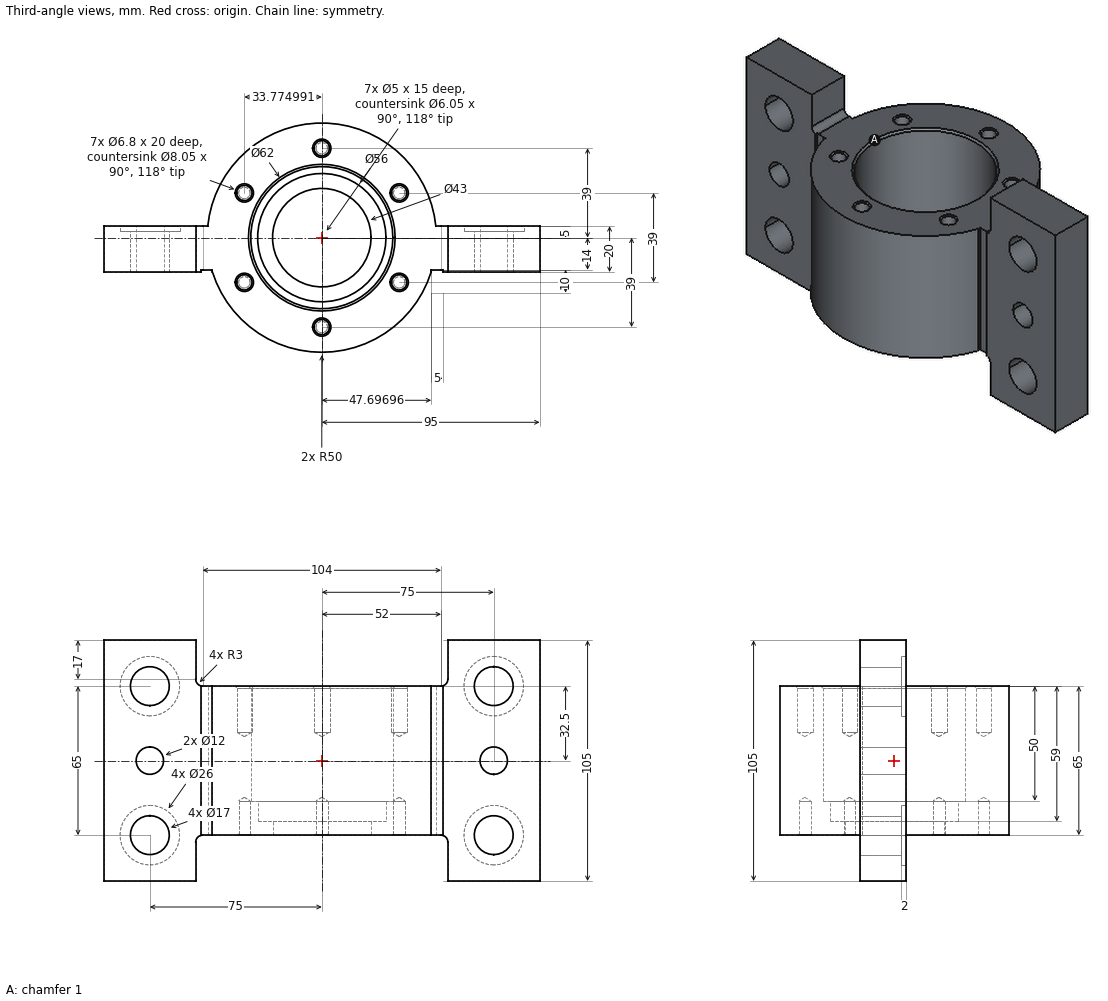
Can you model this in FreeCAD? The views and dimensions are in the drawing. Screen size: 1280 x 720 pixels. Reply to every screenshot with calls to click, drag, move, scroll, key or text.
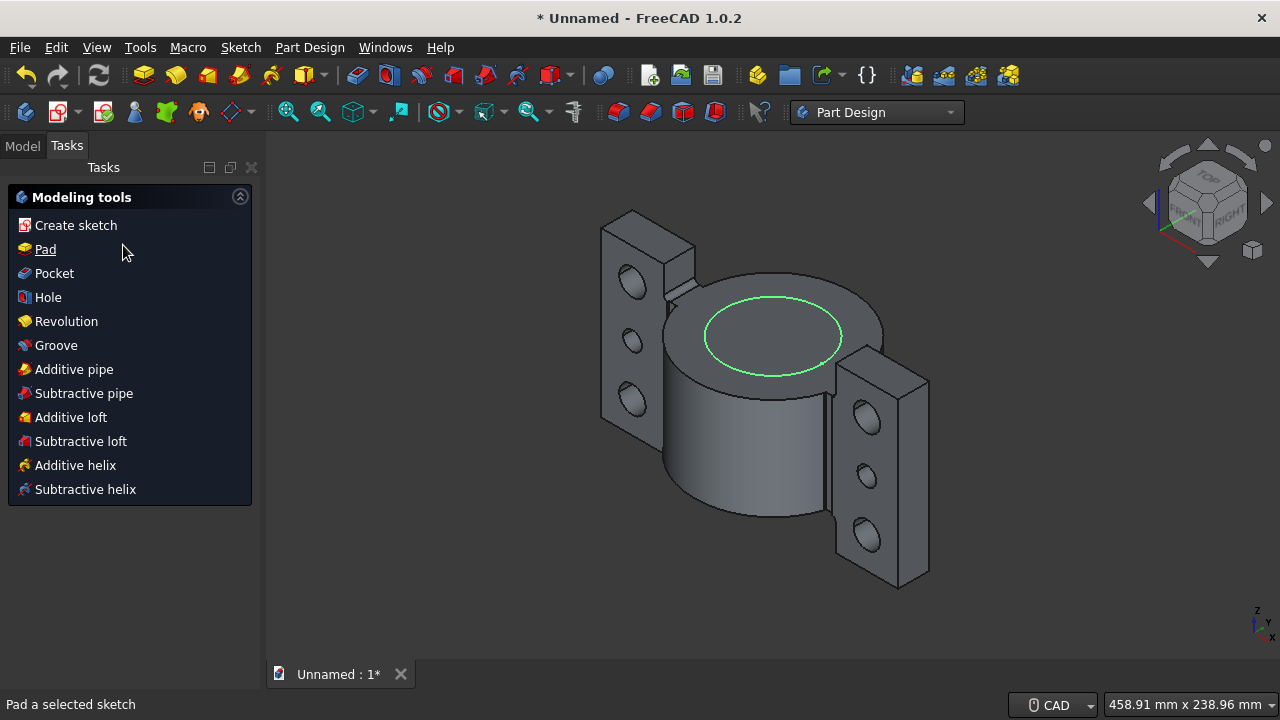
click(358, 76)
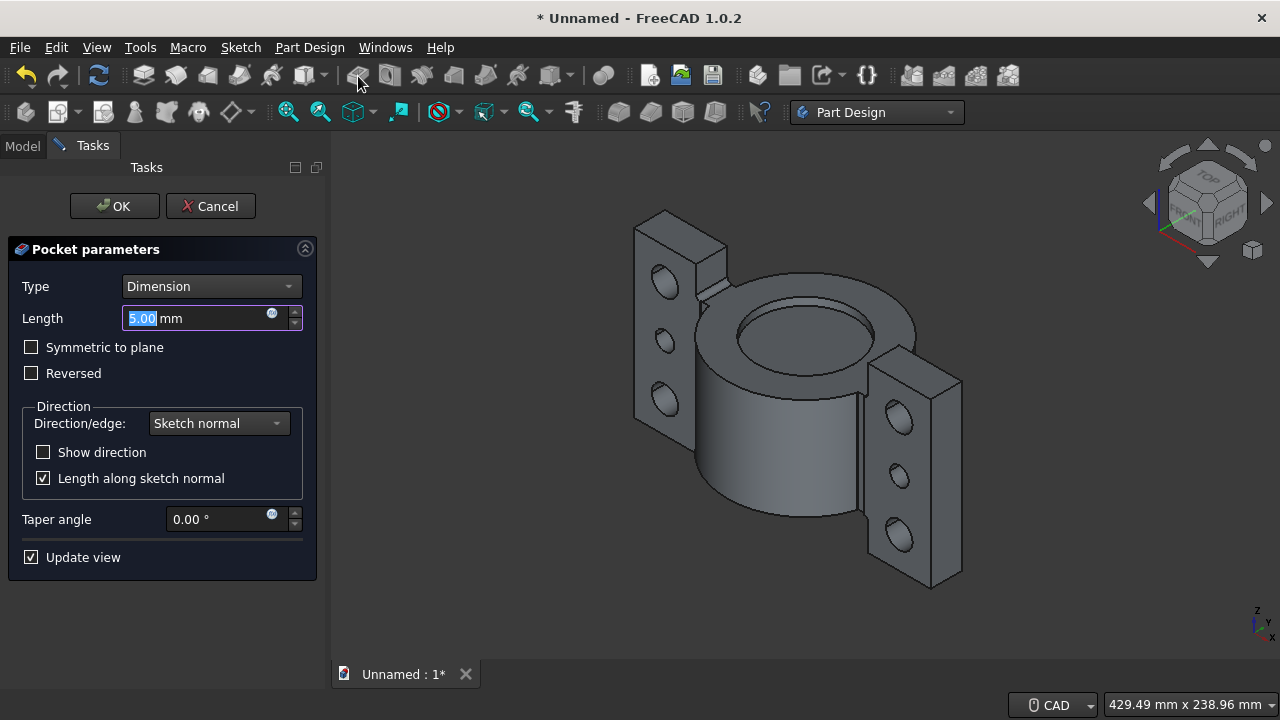
text(50)
key(Tab)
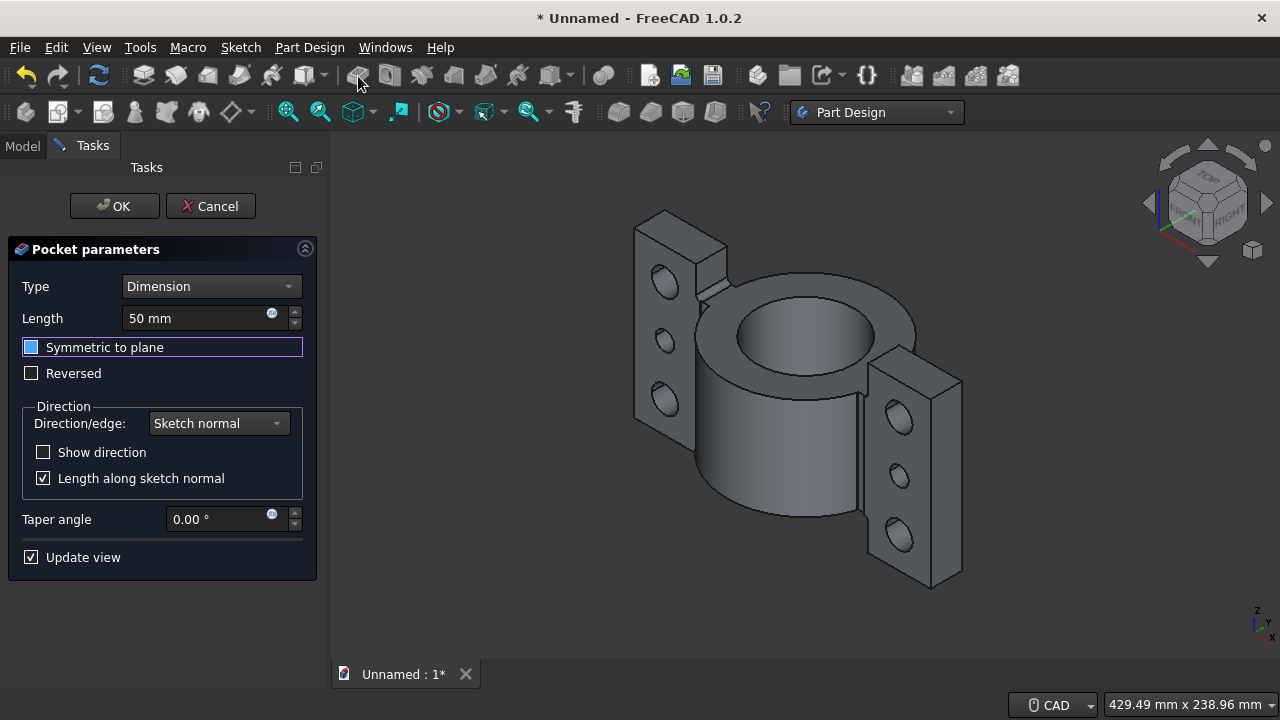
click(115, 206)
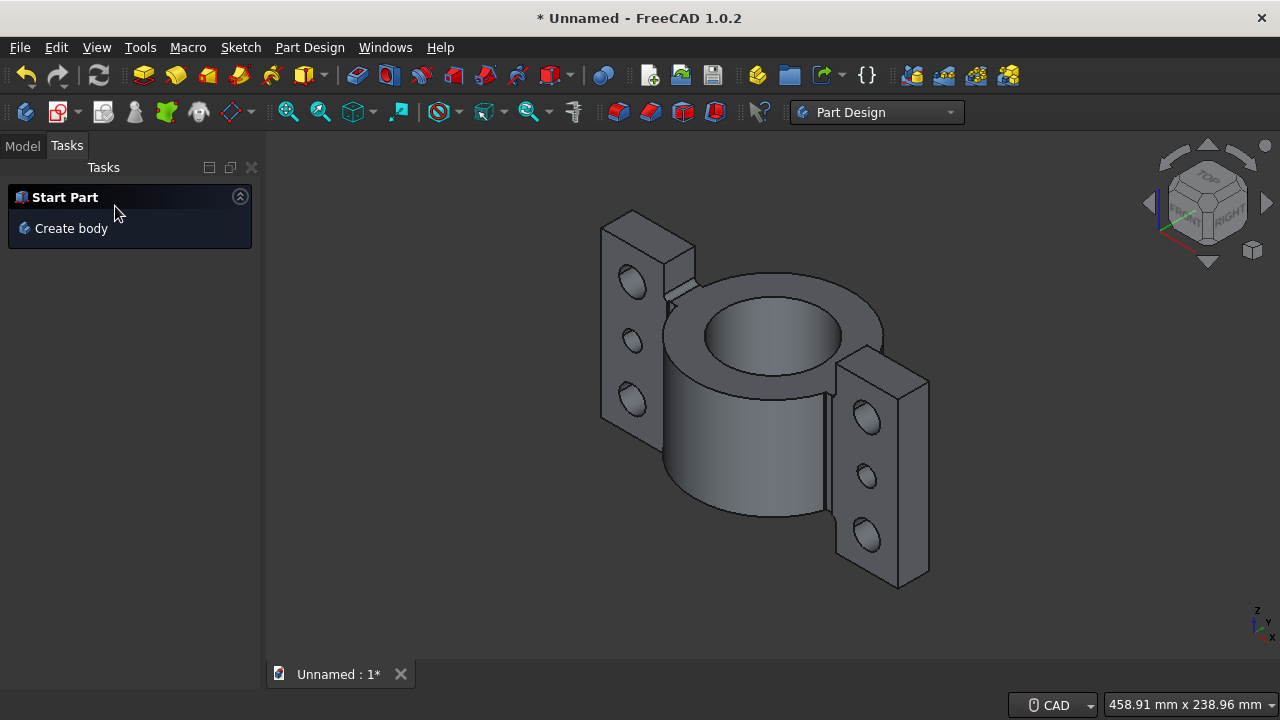
click(771, 283)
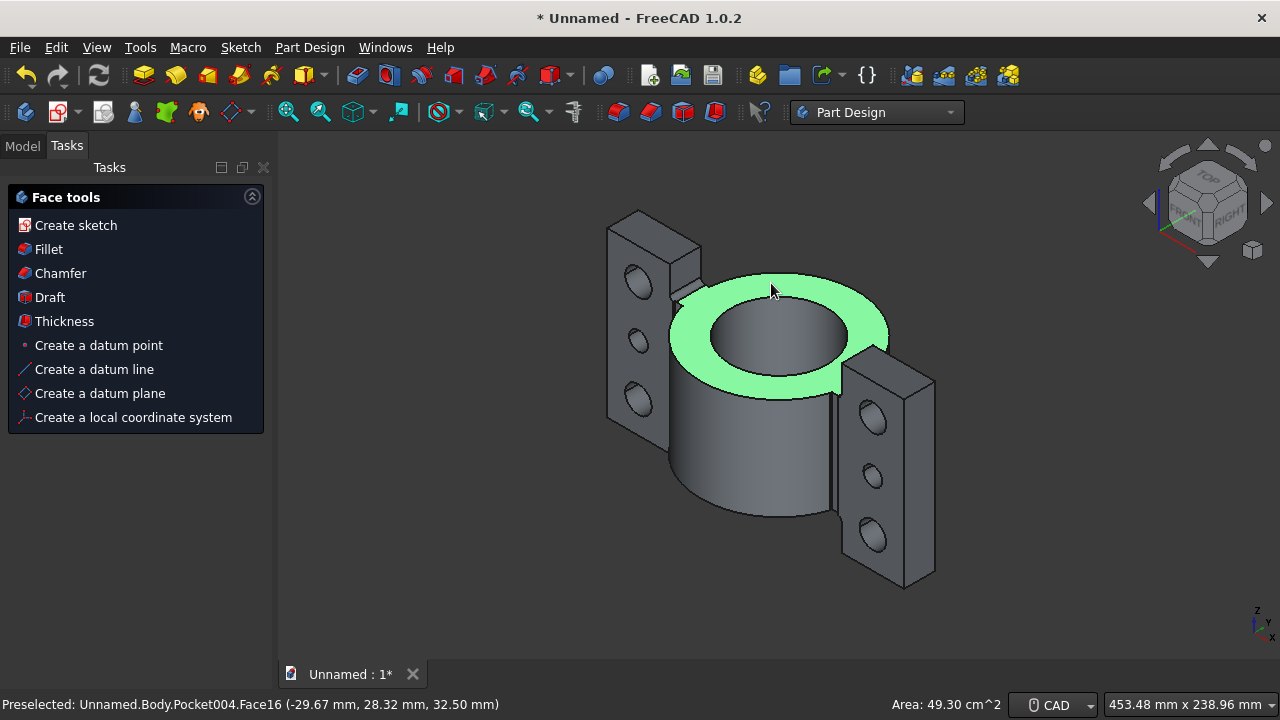
click(58, 112)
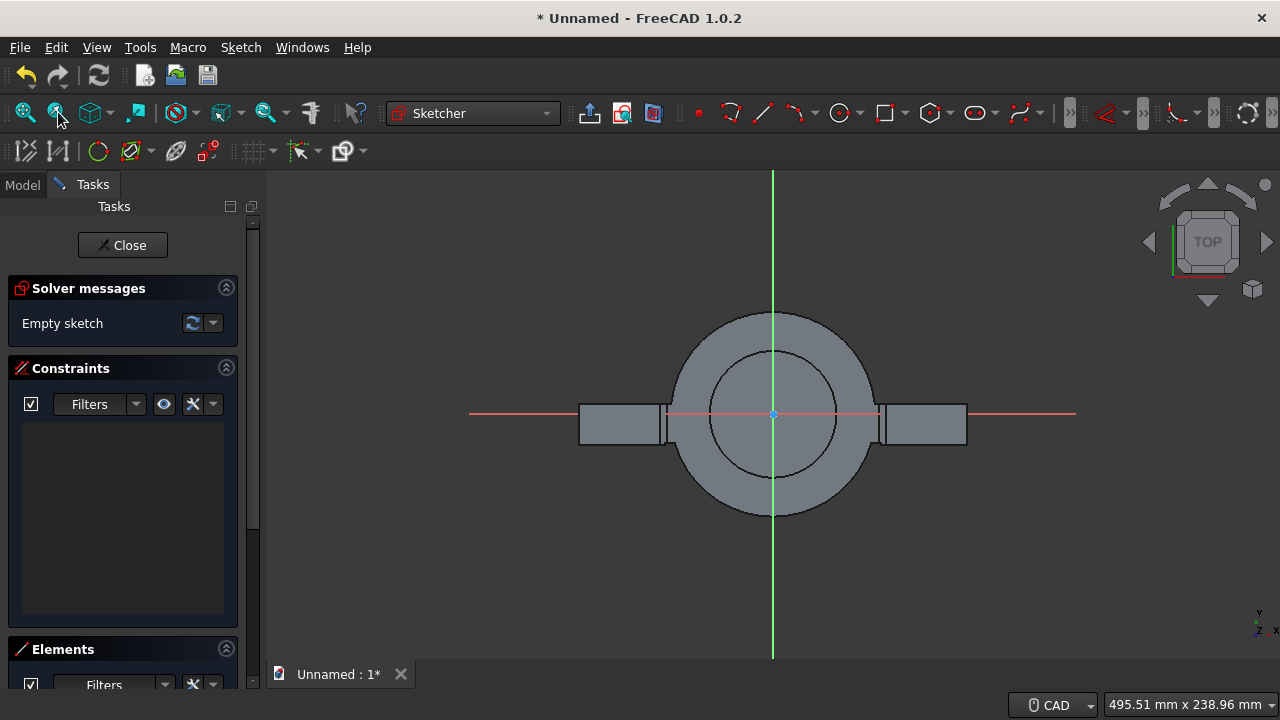
scroll(813, 414, up, 5)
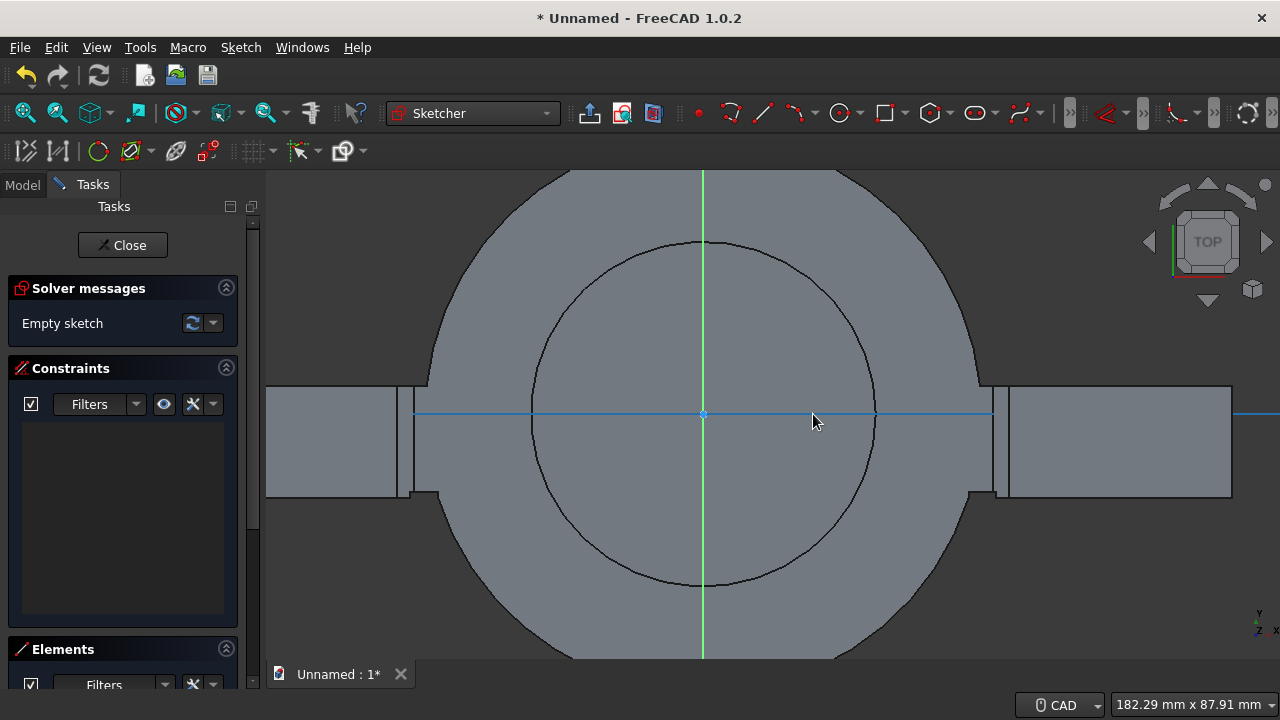
click(840, 114)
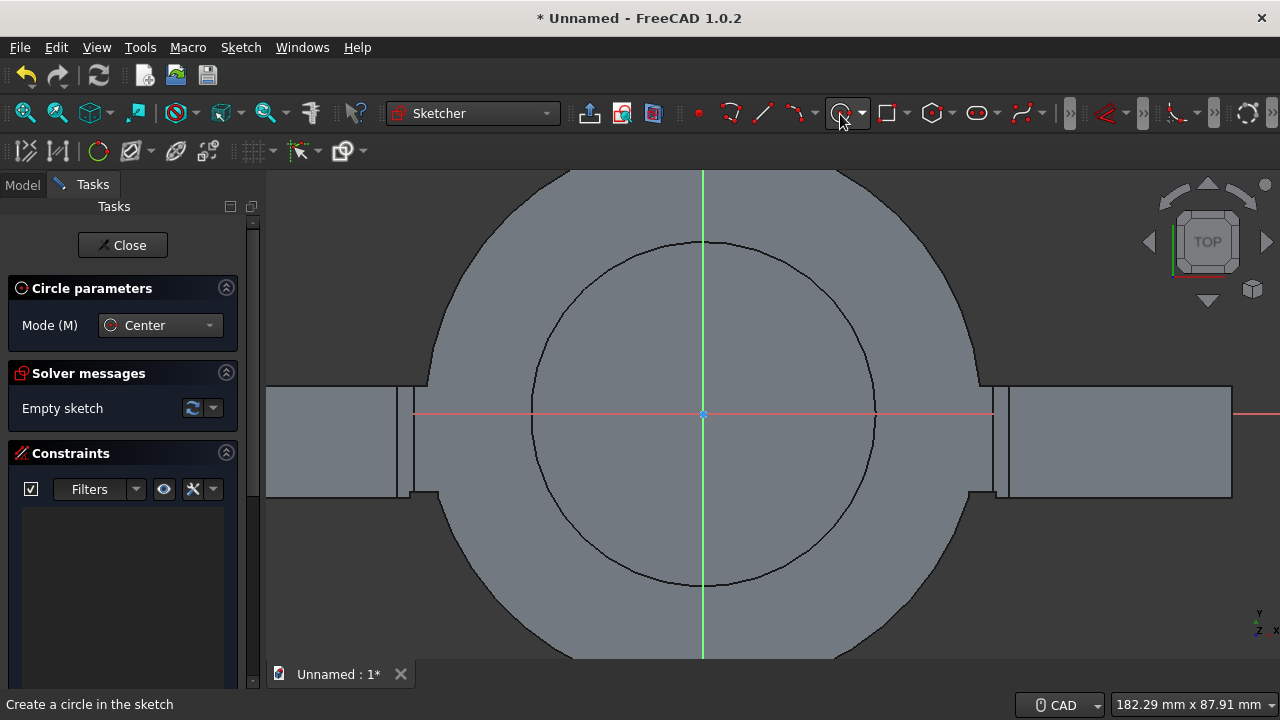
click(703, 414)
click(813, 304)
key(Escape)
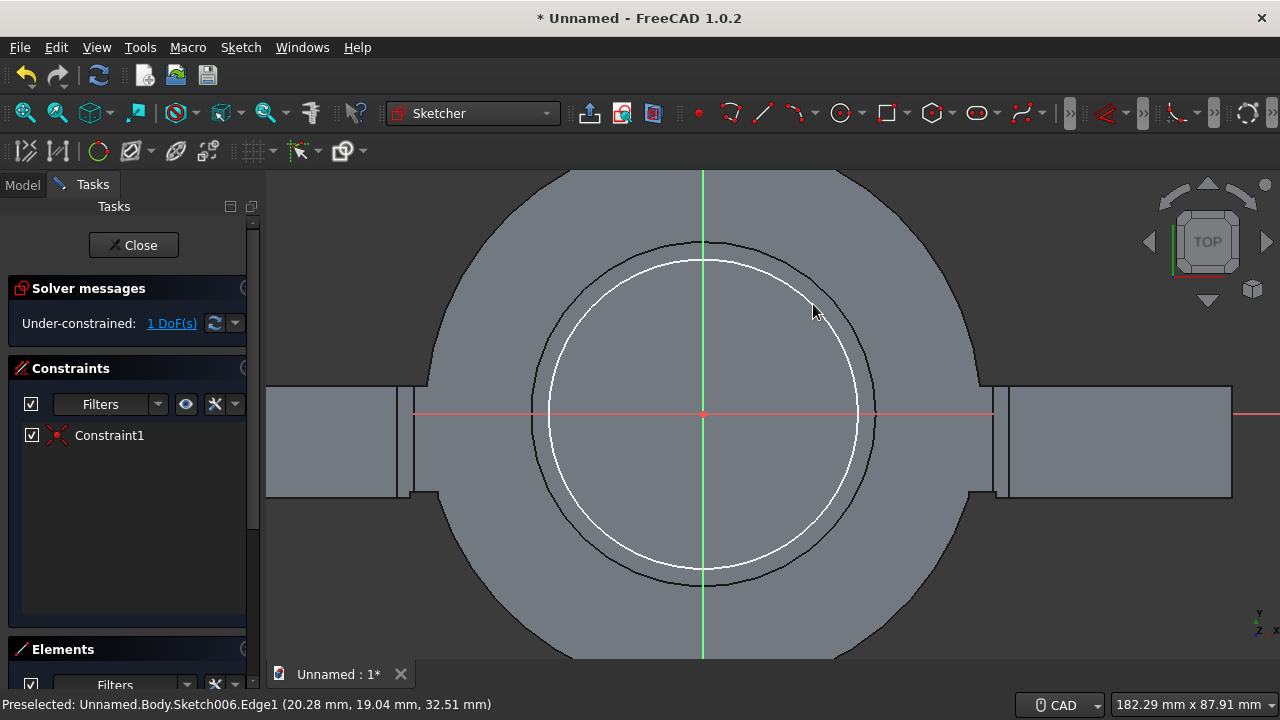
click(1106, 114)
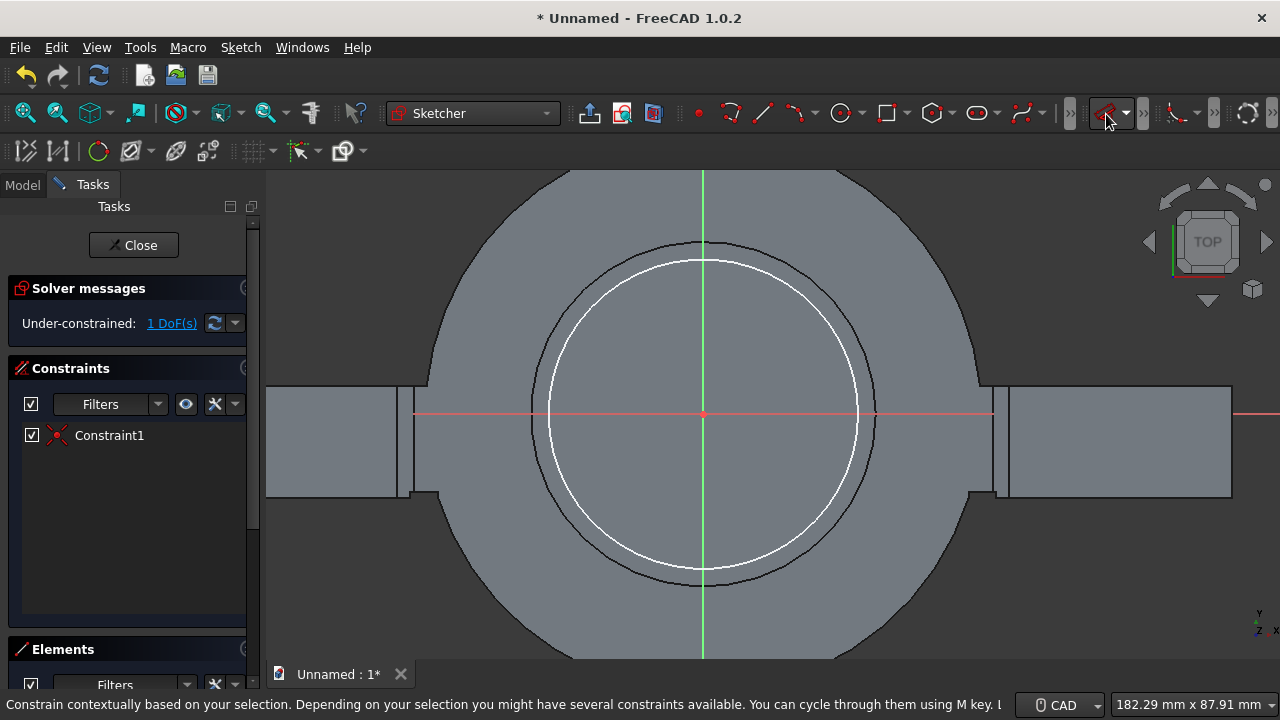
click(812, 304)
click(834, 281)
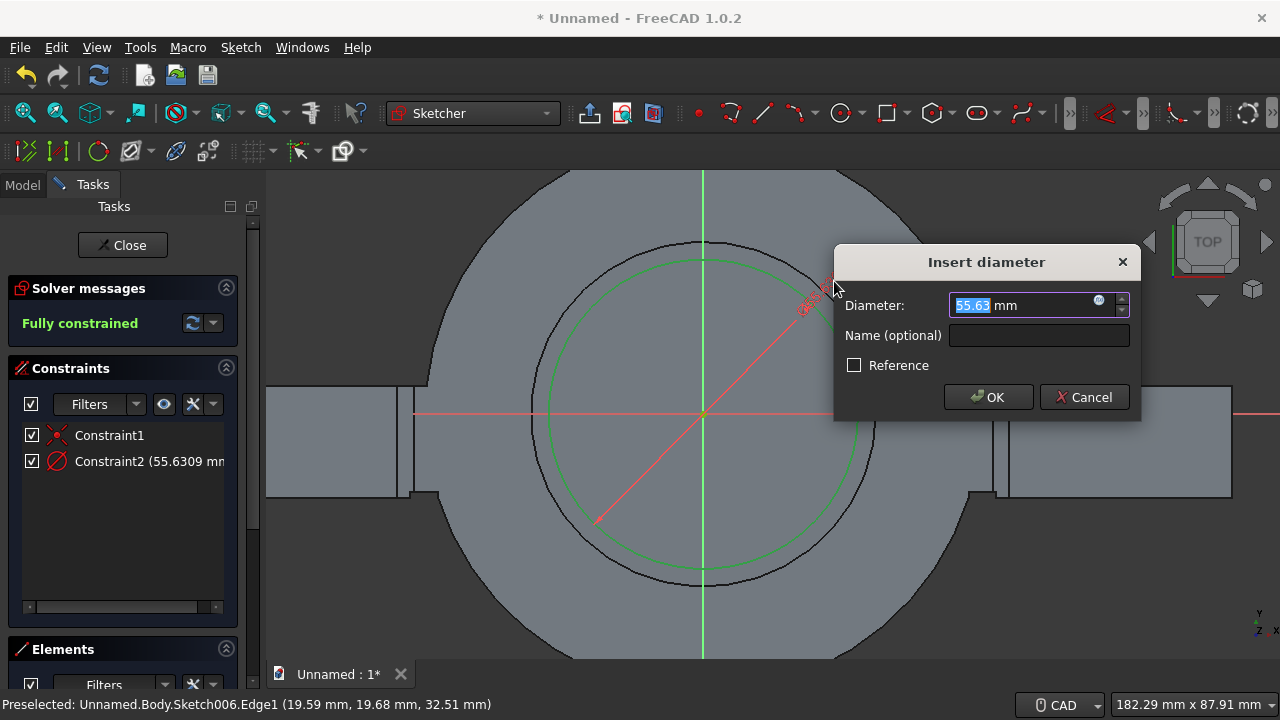
text(56)
key(Return)
key(Escape)